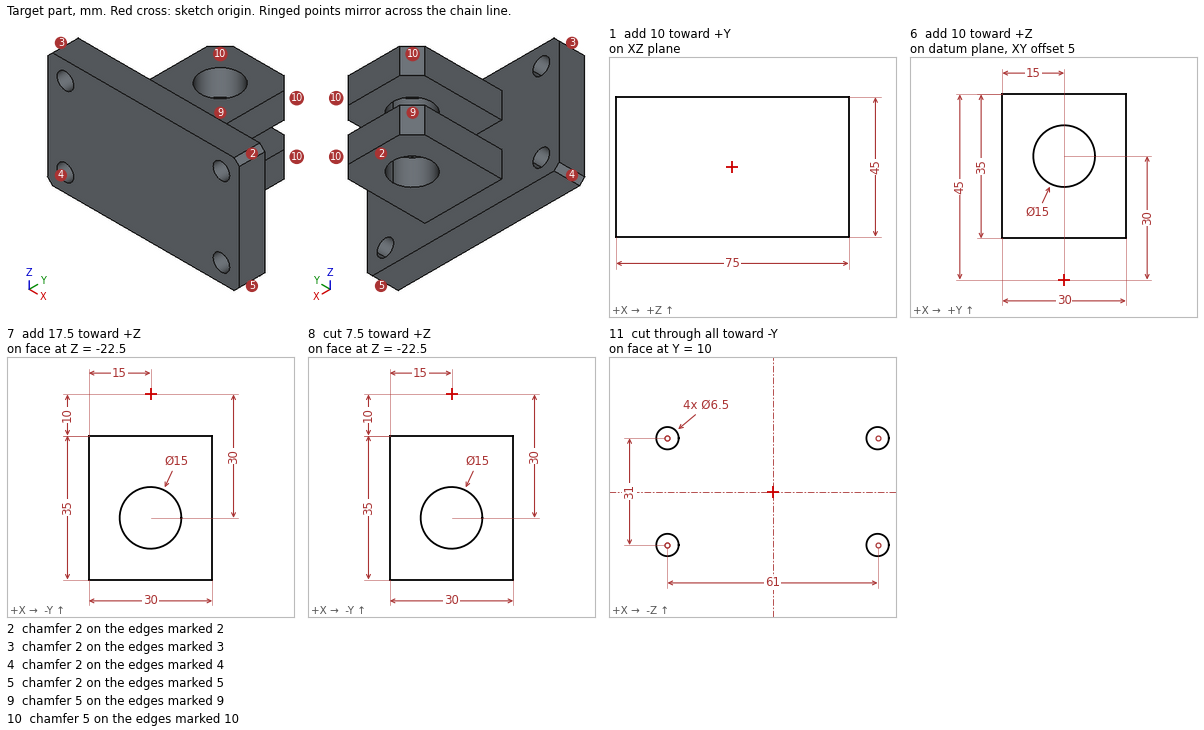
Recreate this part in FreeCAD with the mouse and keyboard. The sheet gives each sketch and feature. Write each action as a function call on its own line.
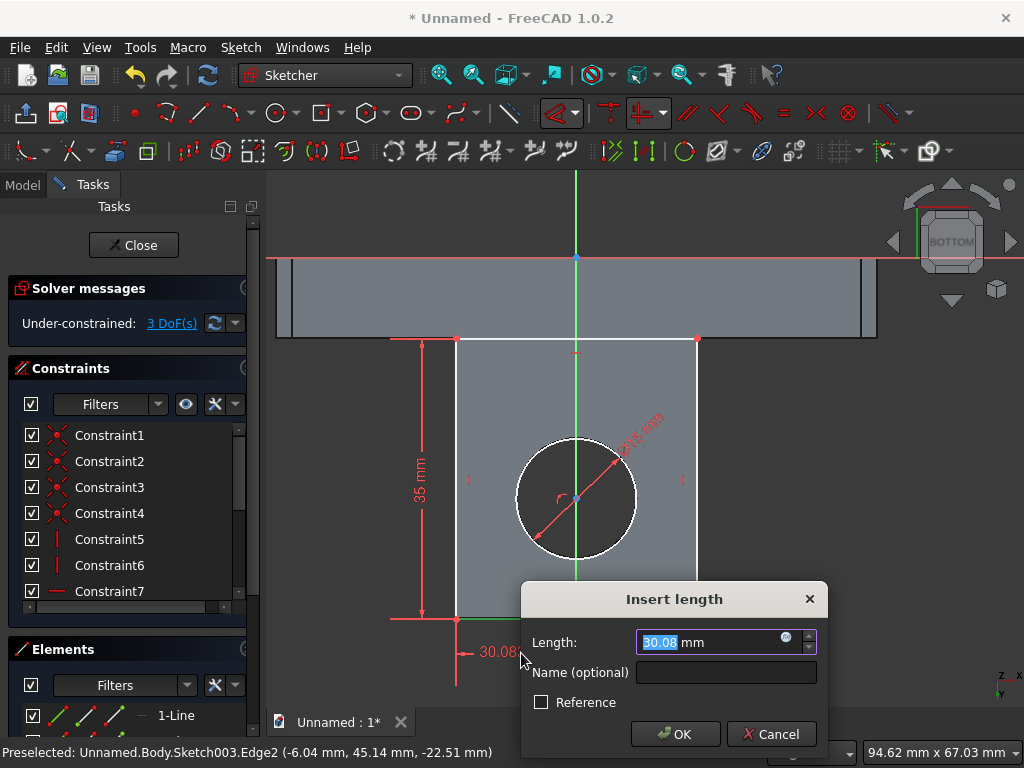
text(30)
key(Return)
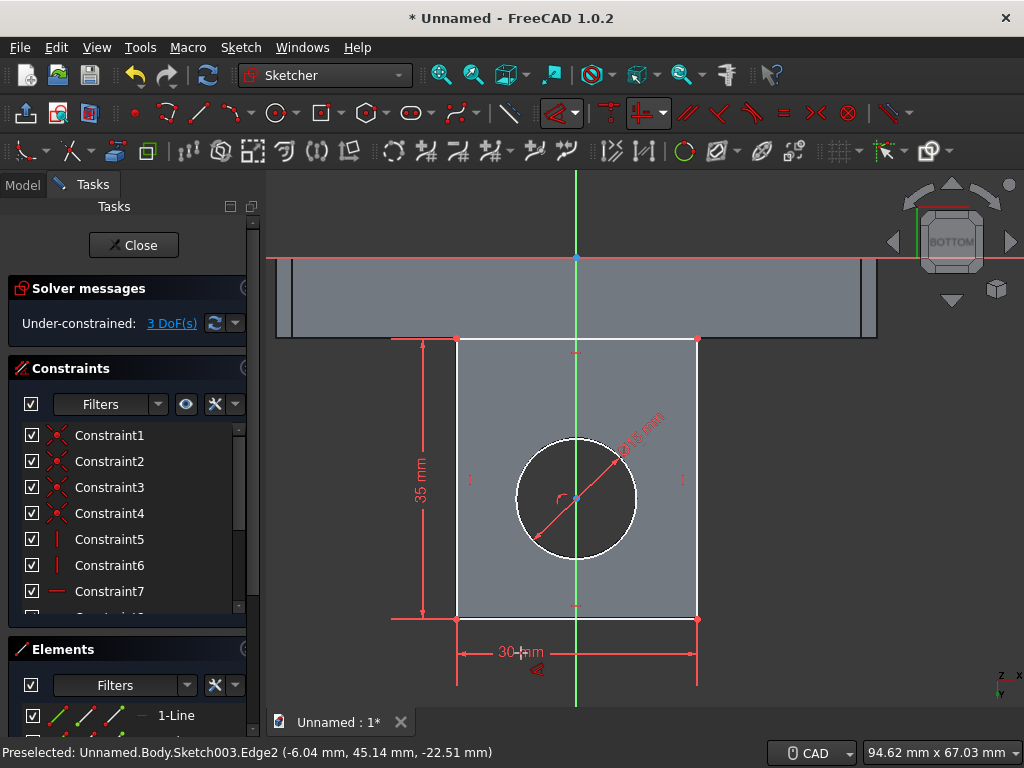
click(576, 499)
click(610, 378)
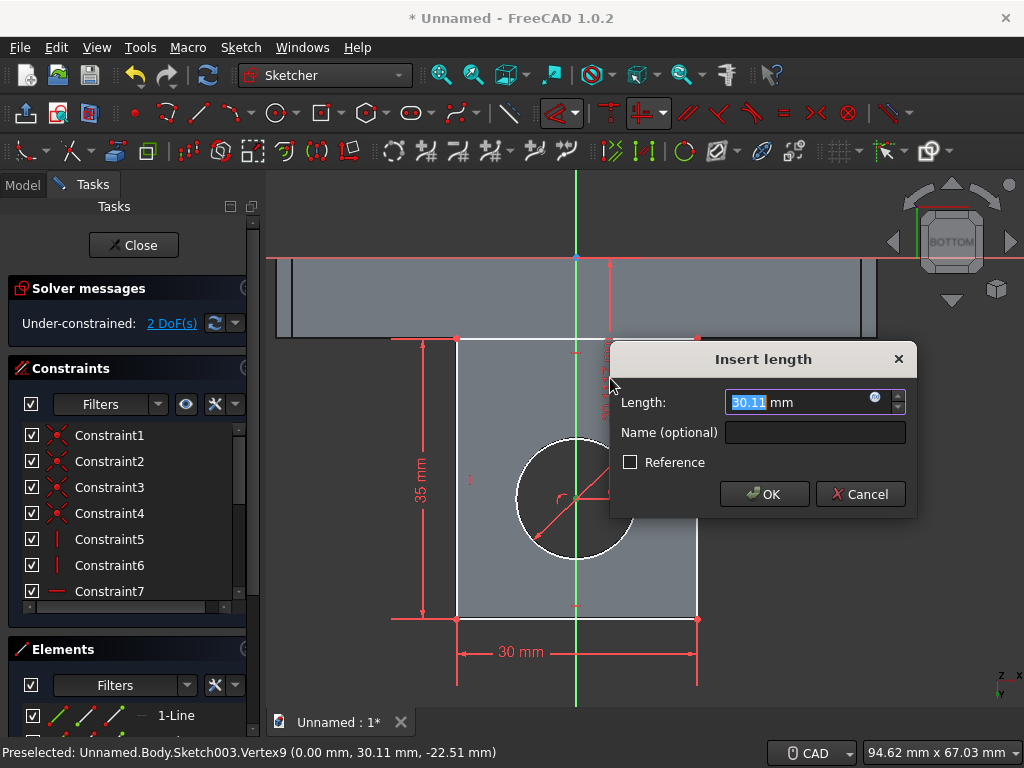
text(30)
key(Return)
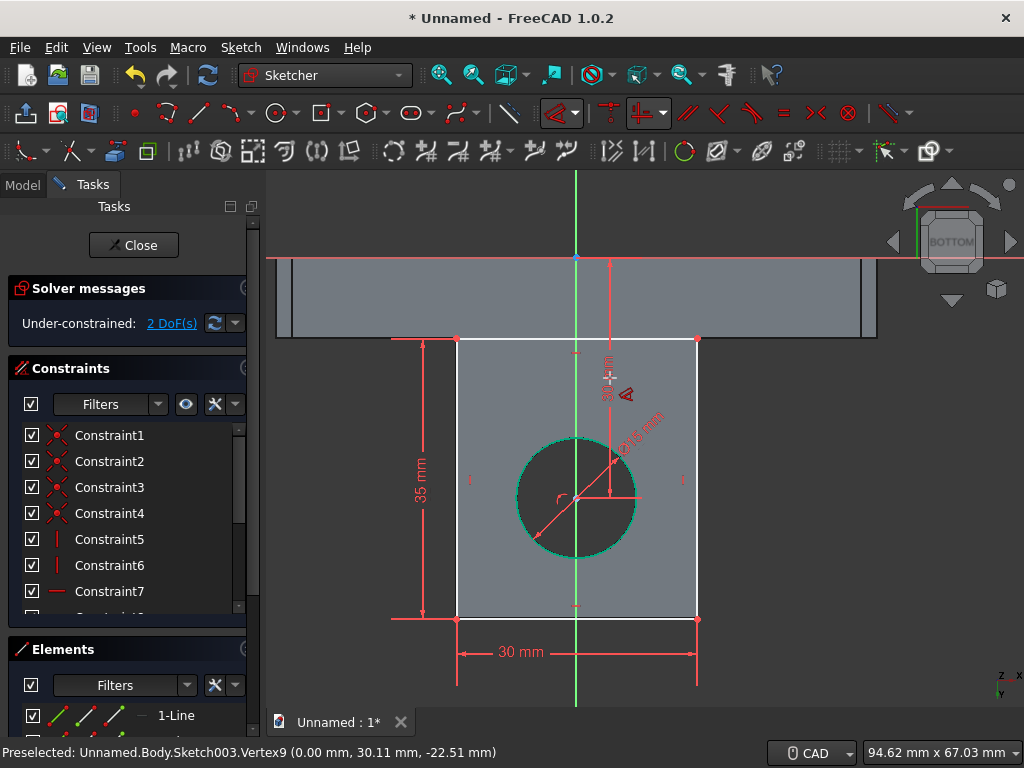
click(457, 339)
click(517, 224)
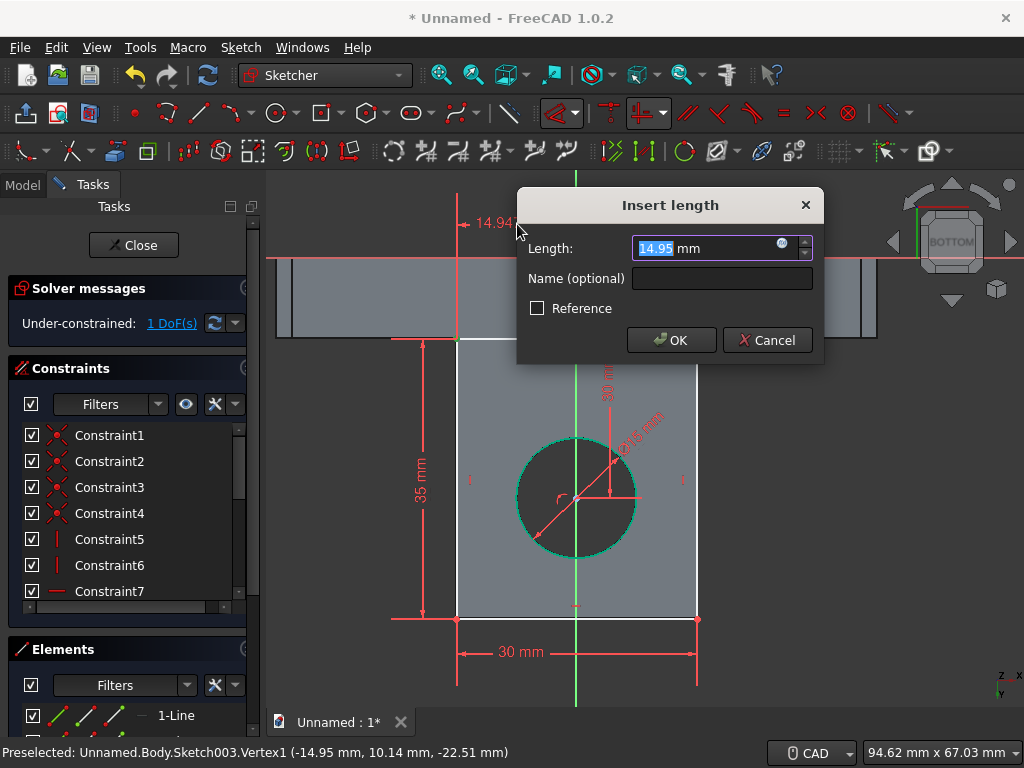
text(15)
key(Return)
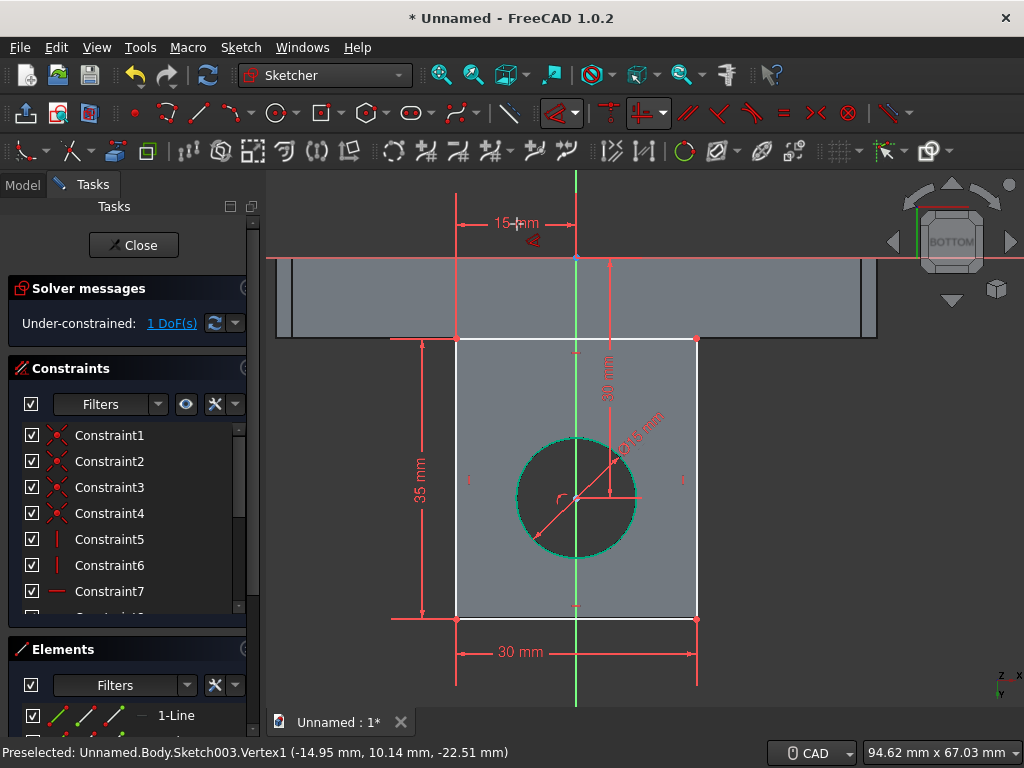
click(456, 339)
click(422, 298)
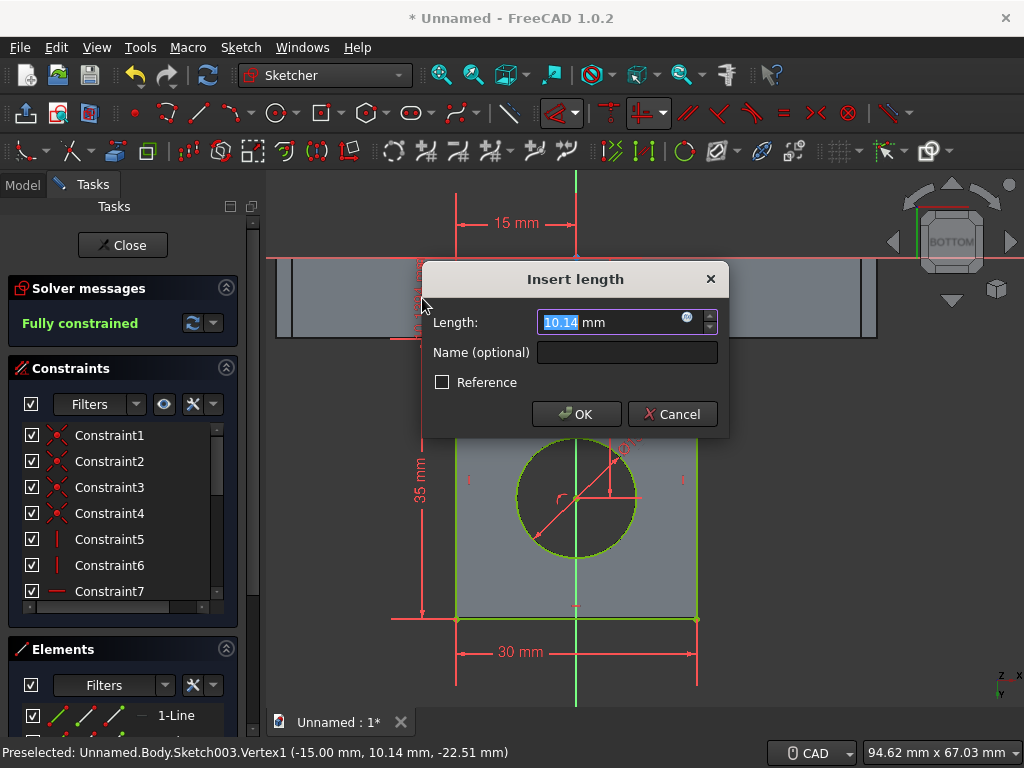
text(10)
key(Return)
key(Escape)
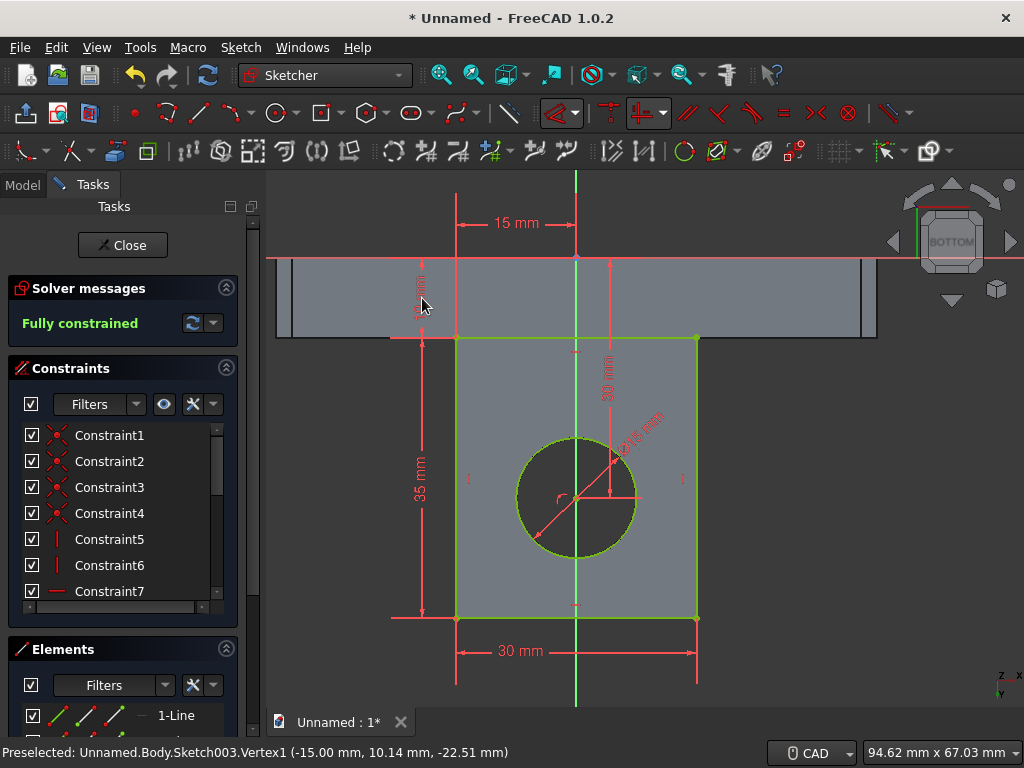
click(123, 245)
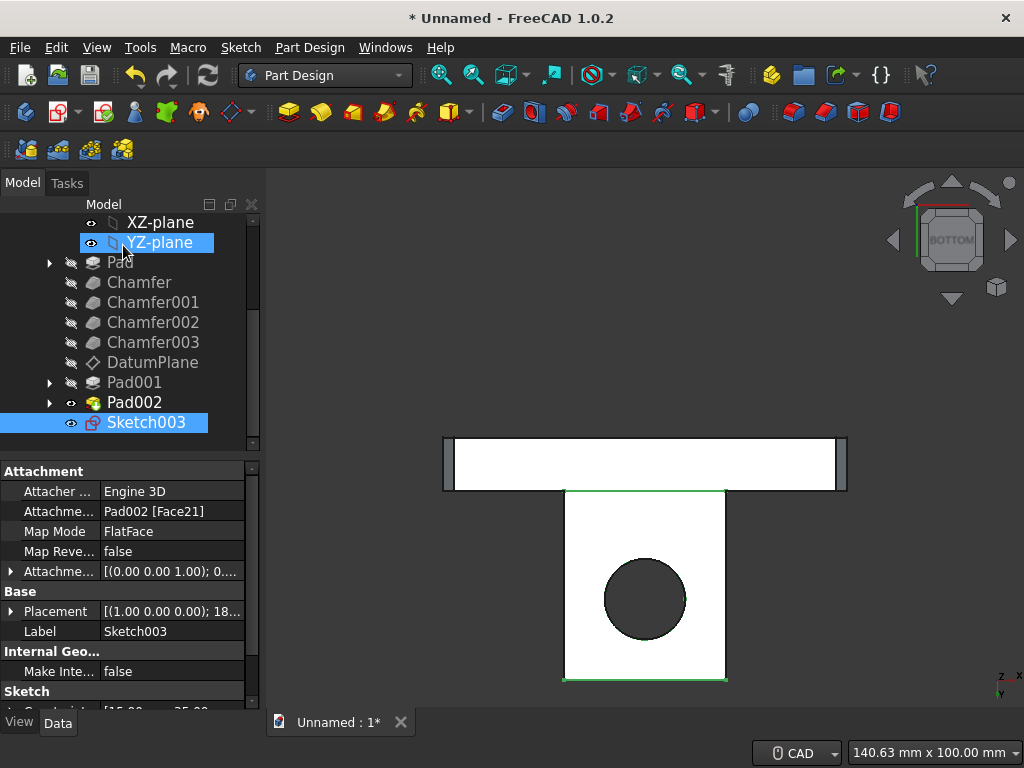
click(504, 112)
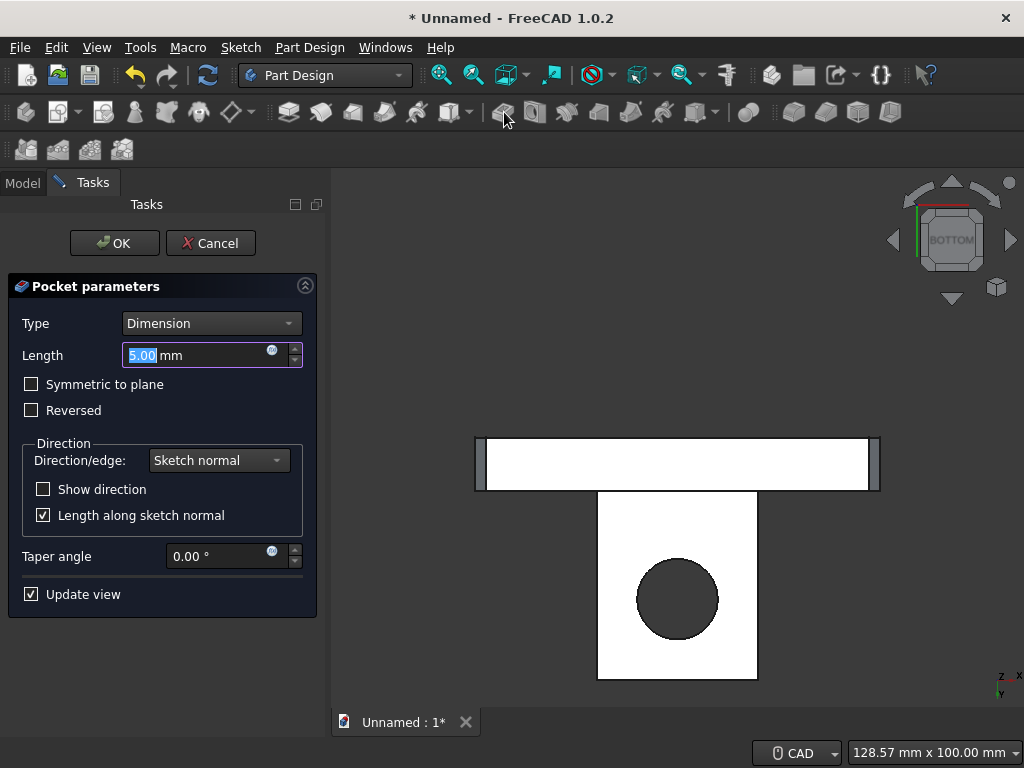
text(7.5)
key(Tab)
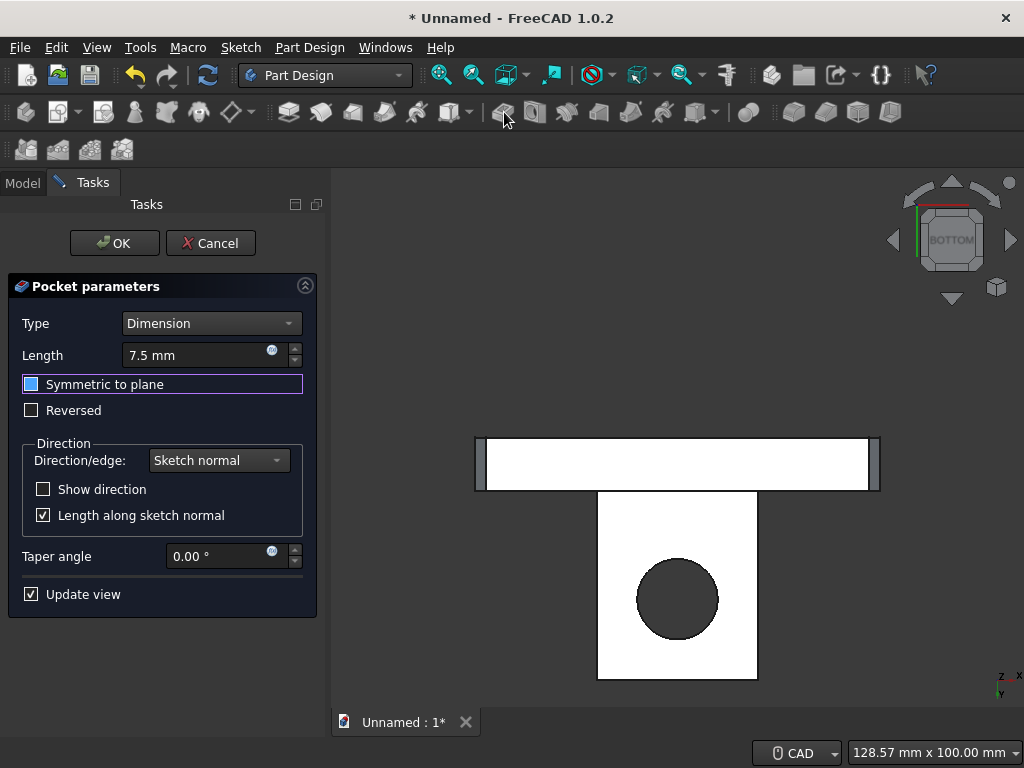
click(115, 243)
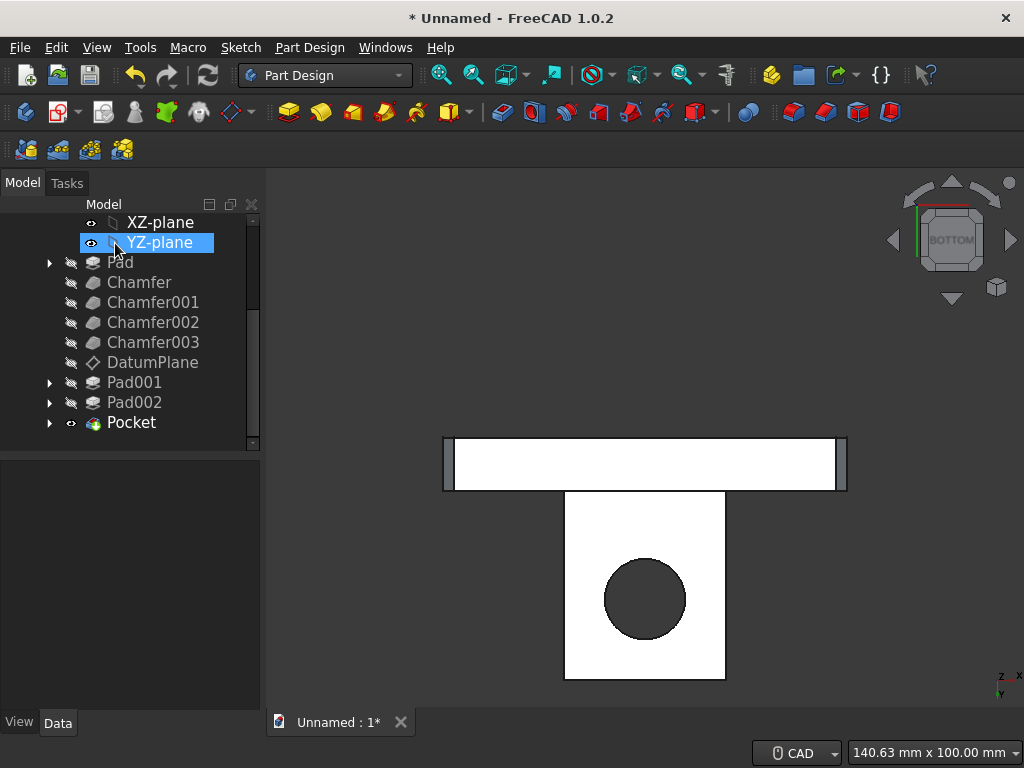
key(0)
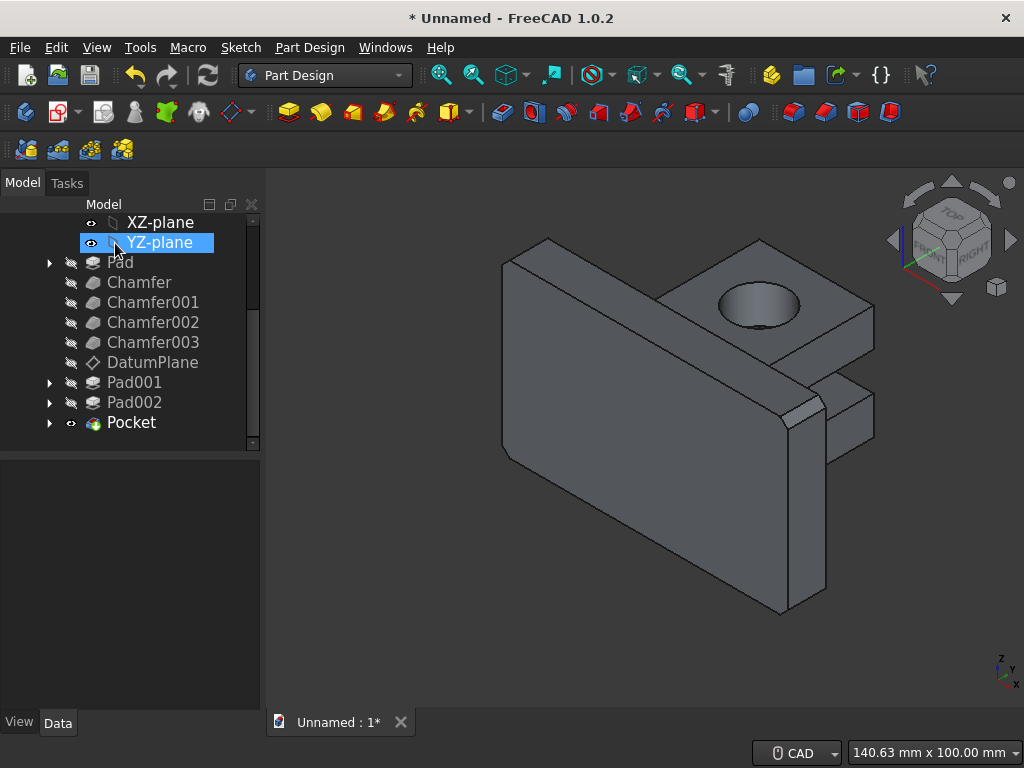
key(v)
key(f)